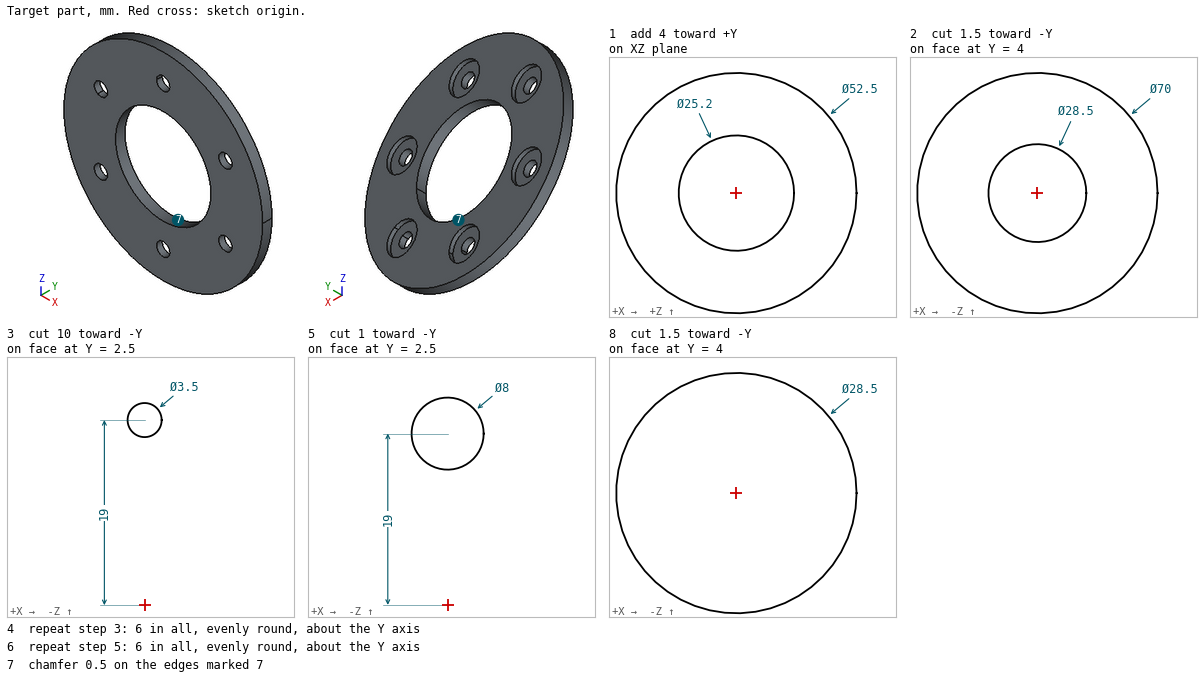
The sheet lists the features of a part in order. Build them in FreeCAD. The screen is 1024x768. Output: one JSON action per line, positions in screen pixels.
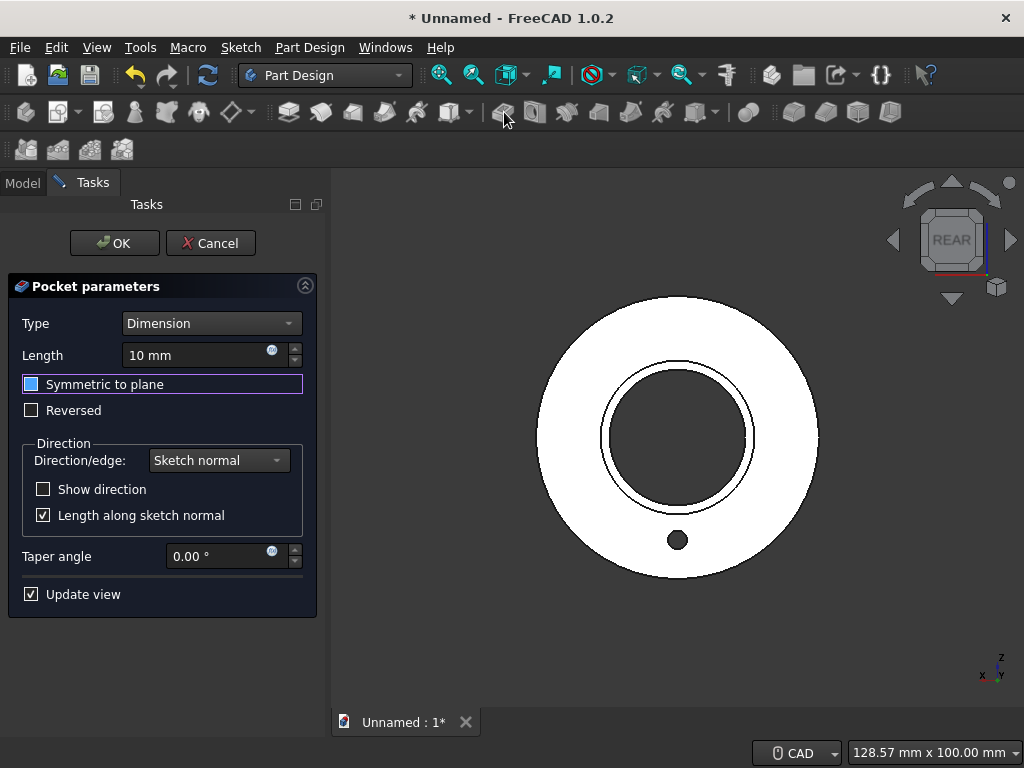
{"action": "left_click", "coordinate": [115, 243]}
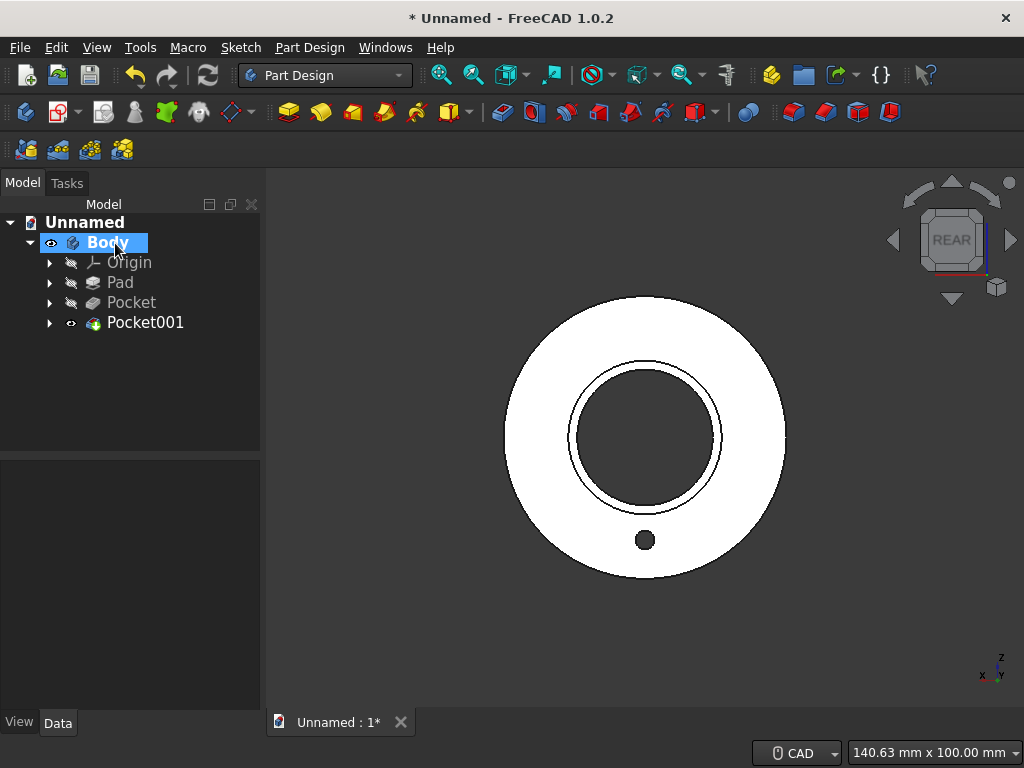
{"action": "left_click", "coordinate": [116, 323]}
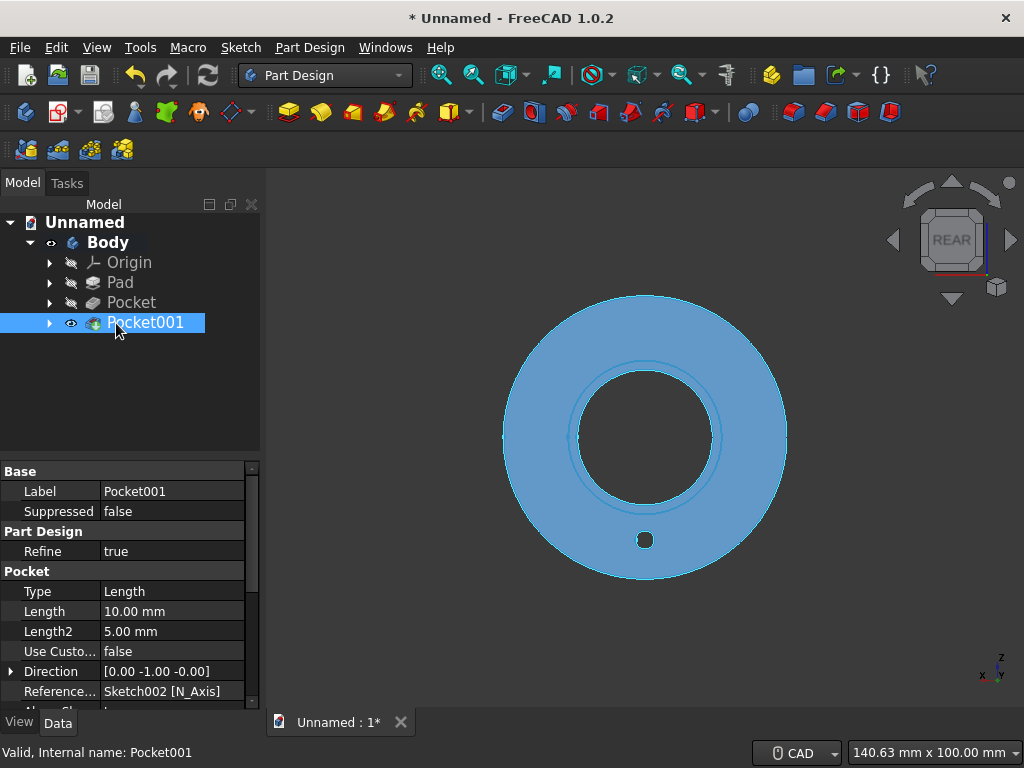
{"action": "left_click", "coordinate": [90, 150]}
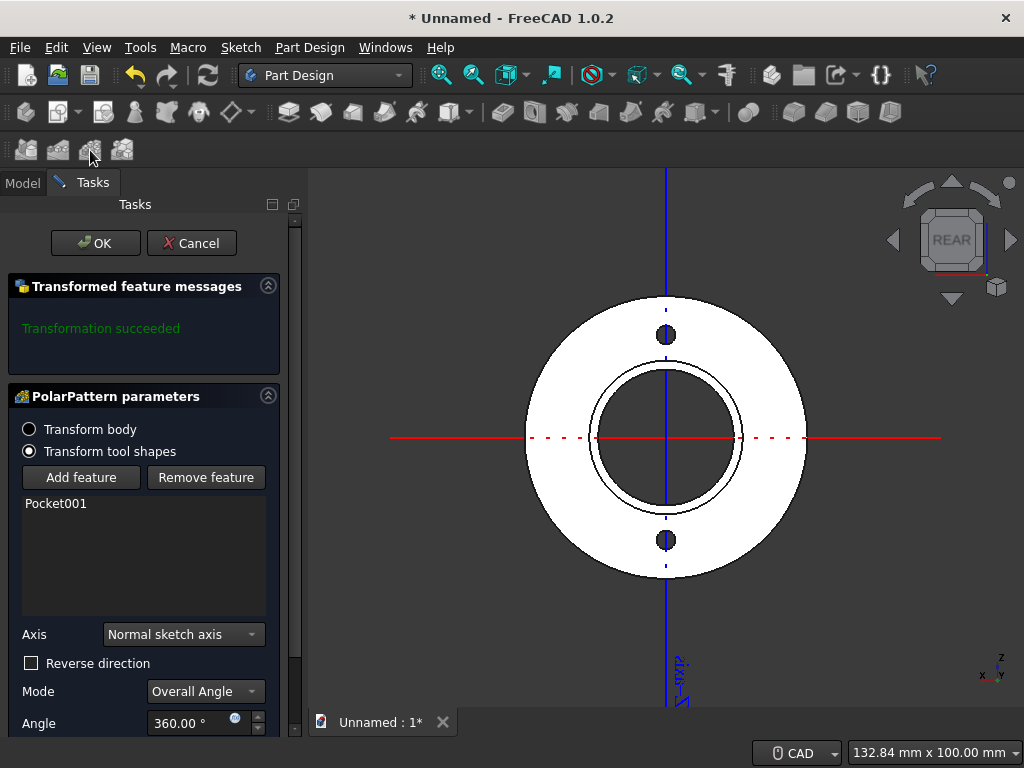
{"action": "left_click", "coordinate": [184, 634]}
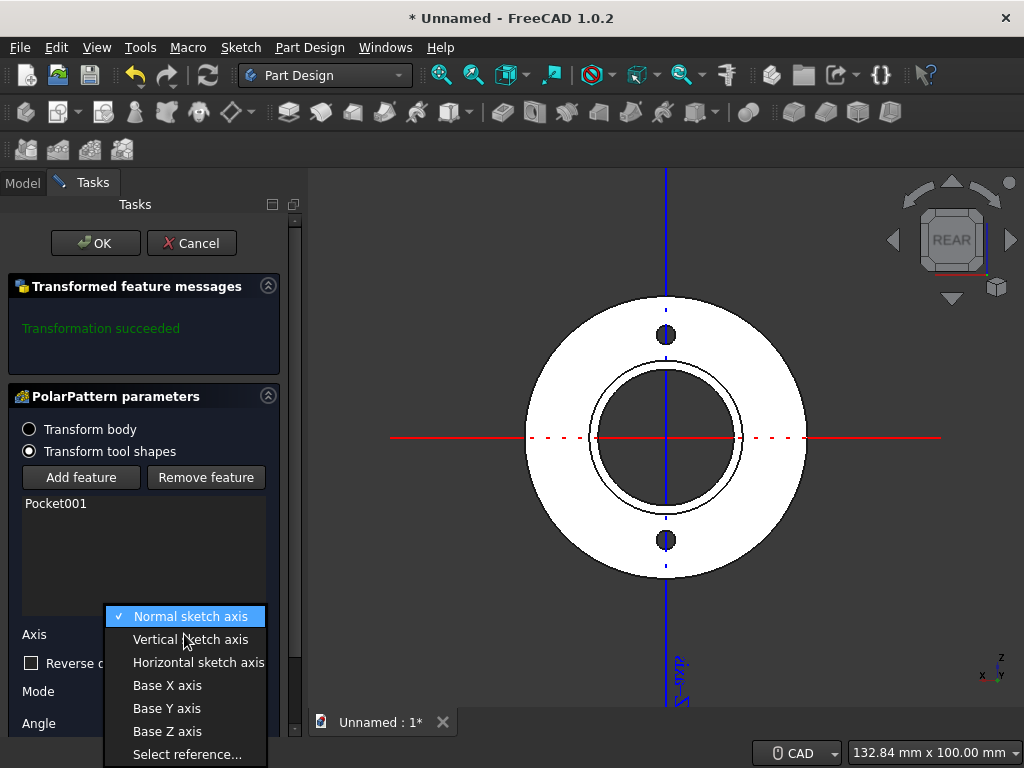
{"action": "left_click", "coordinate": [184, 708]}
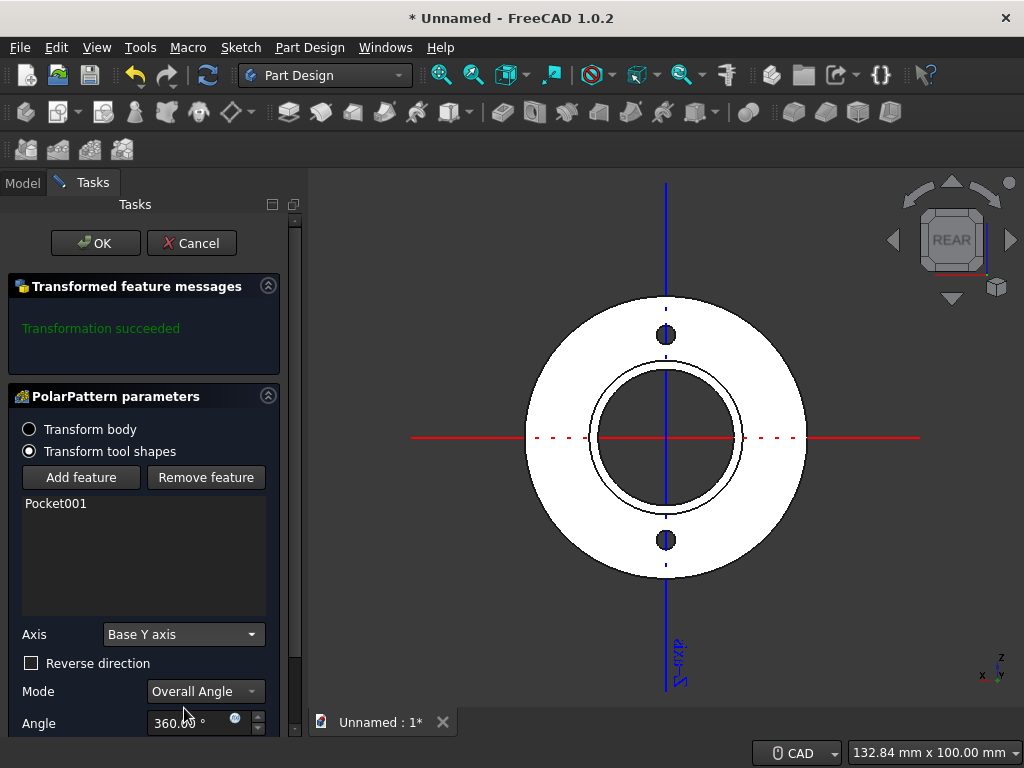
{"action": "scroll", "coordinate": [295, 475], "scroll_direction": "down", "scroll_amount": 2}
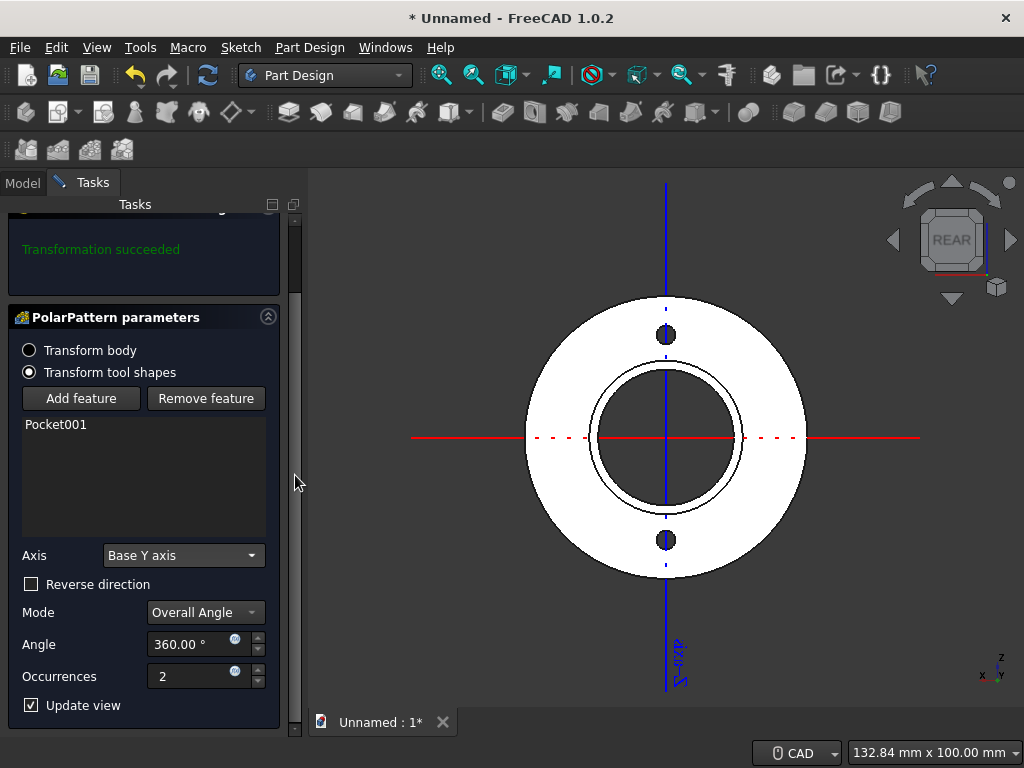
{"action": "triple_click", "coordinate": [198, 676]}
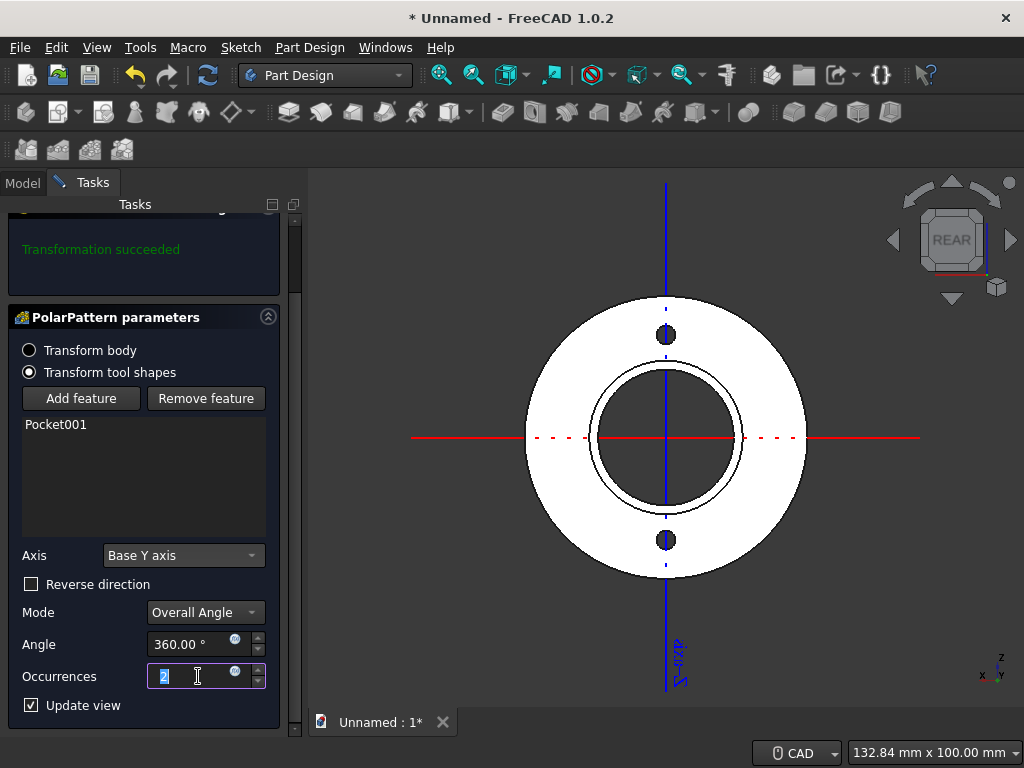
{"action": "type", "text": "6"}
{"action": "key", "text": "Tab"}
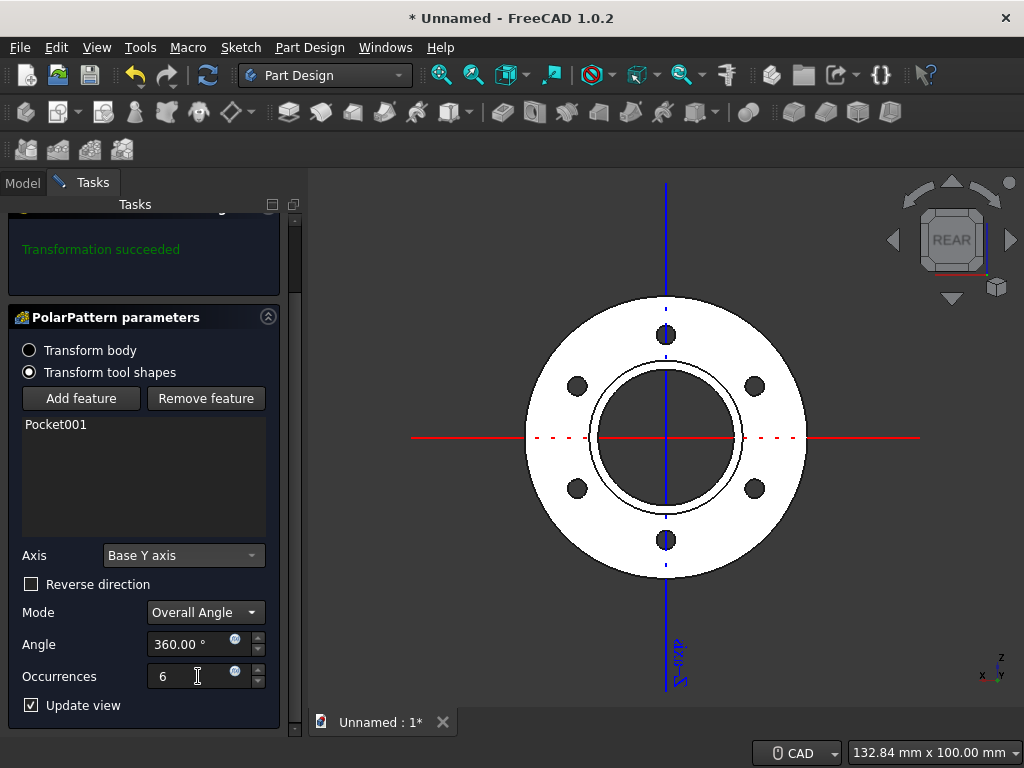
{"action": "scroll", "coordinate": [295, 475], "scroll_direction": "up", "scroll_amount": 3}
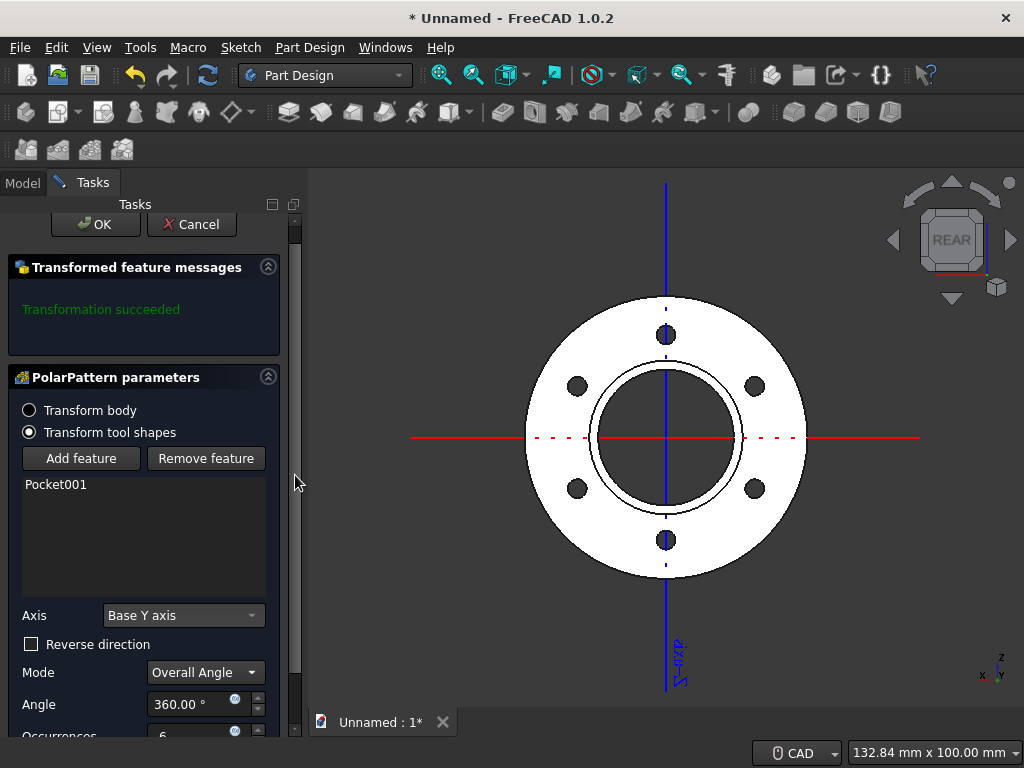
{"action": "left_click", "coordinate": [96, 243]}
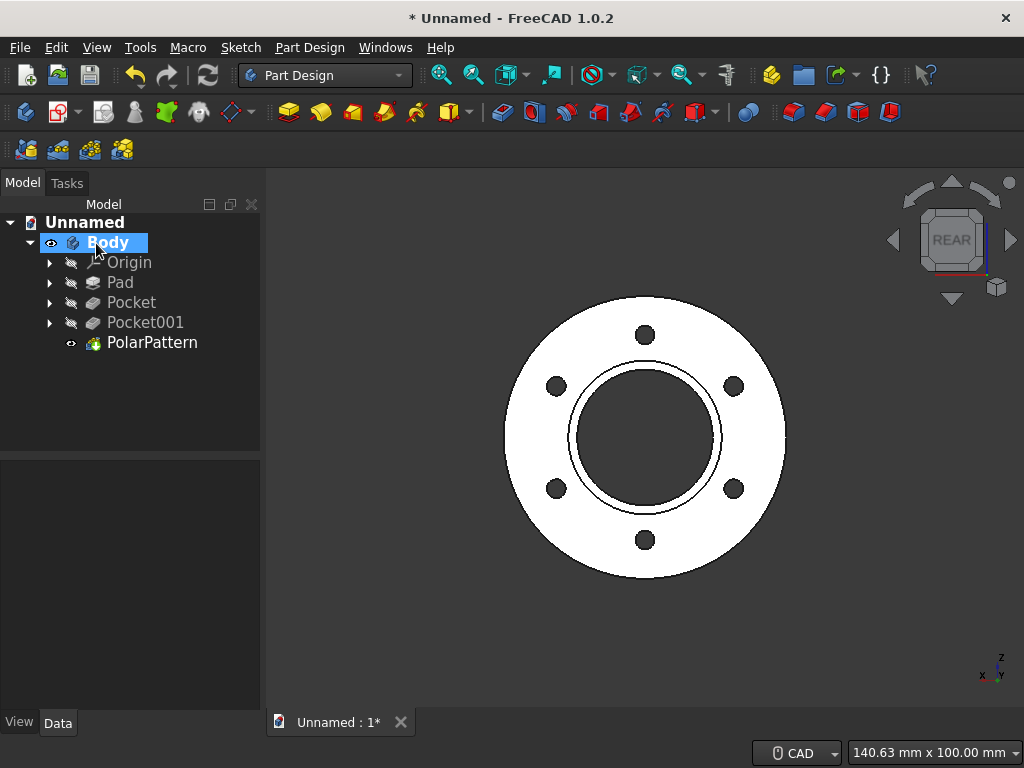
{"action": "left_click", "coordinate": [564, 517]}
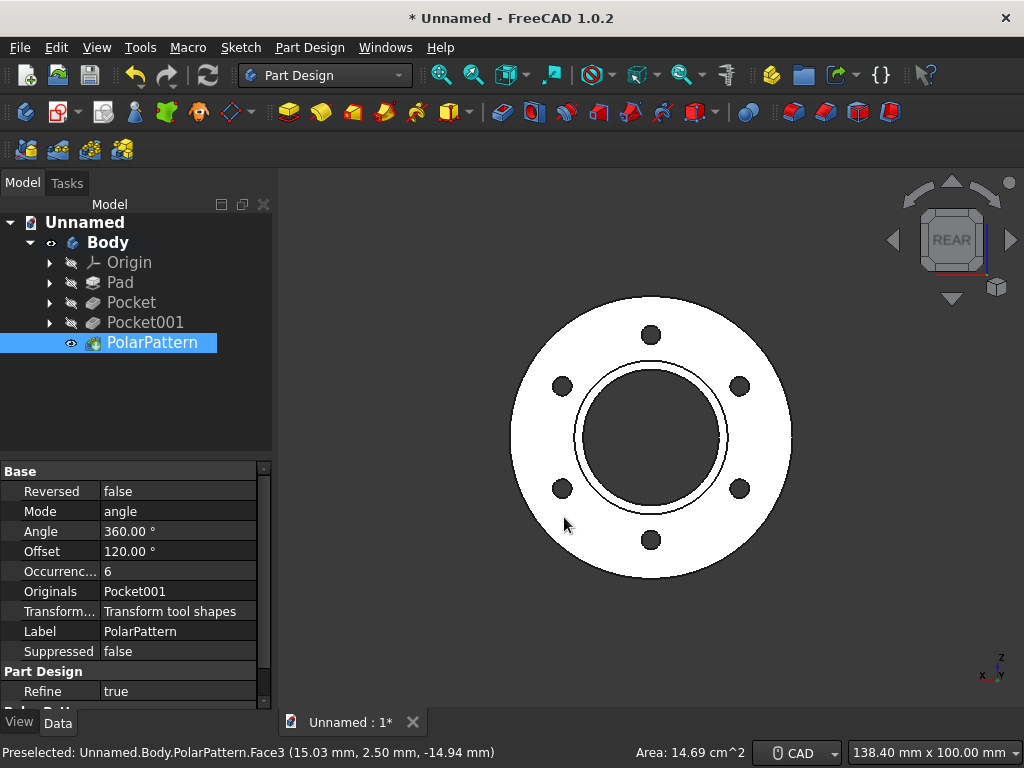
{"action": "left_click", "coordinate": [58, 112]}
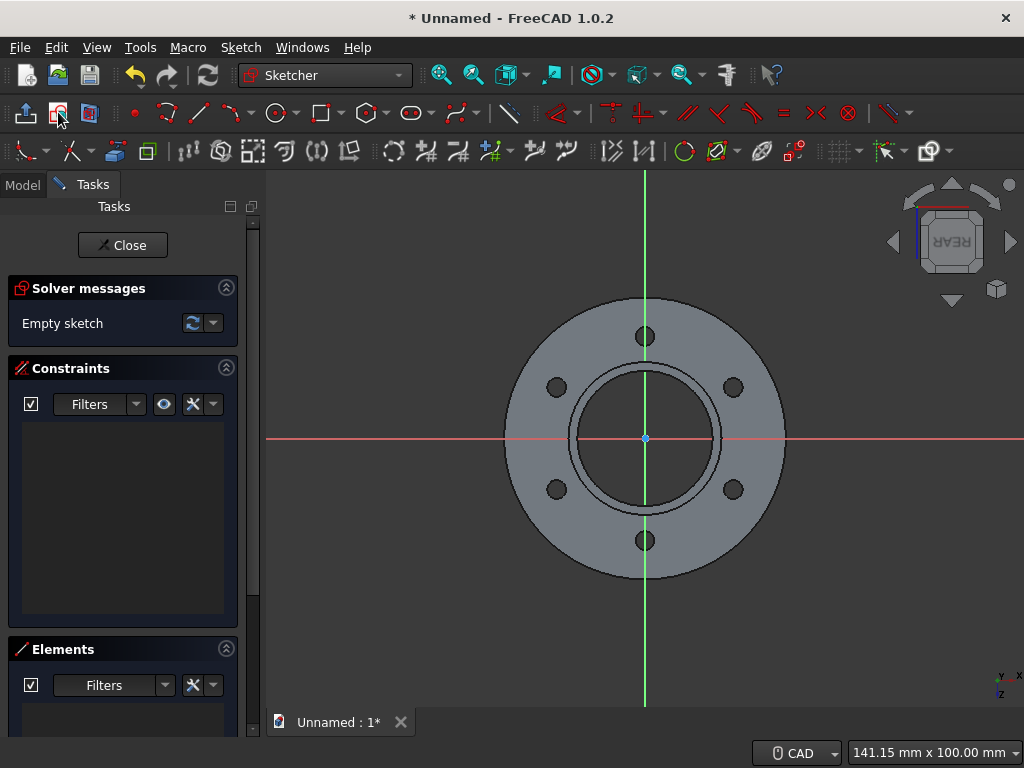
{"action": "scroll", "coordinate": [656, 321], "scroll_direction": "up", "scroll_amount": 10}